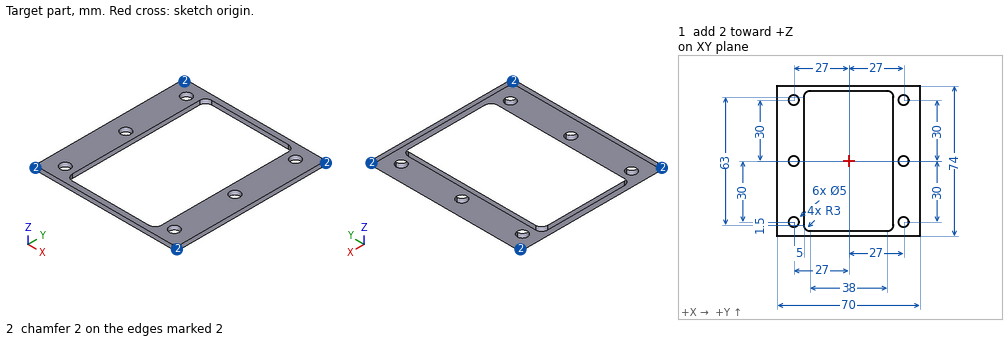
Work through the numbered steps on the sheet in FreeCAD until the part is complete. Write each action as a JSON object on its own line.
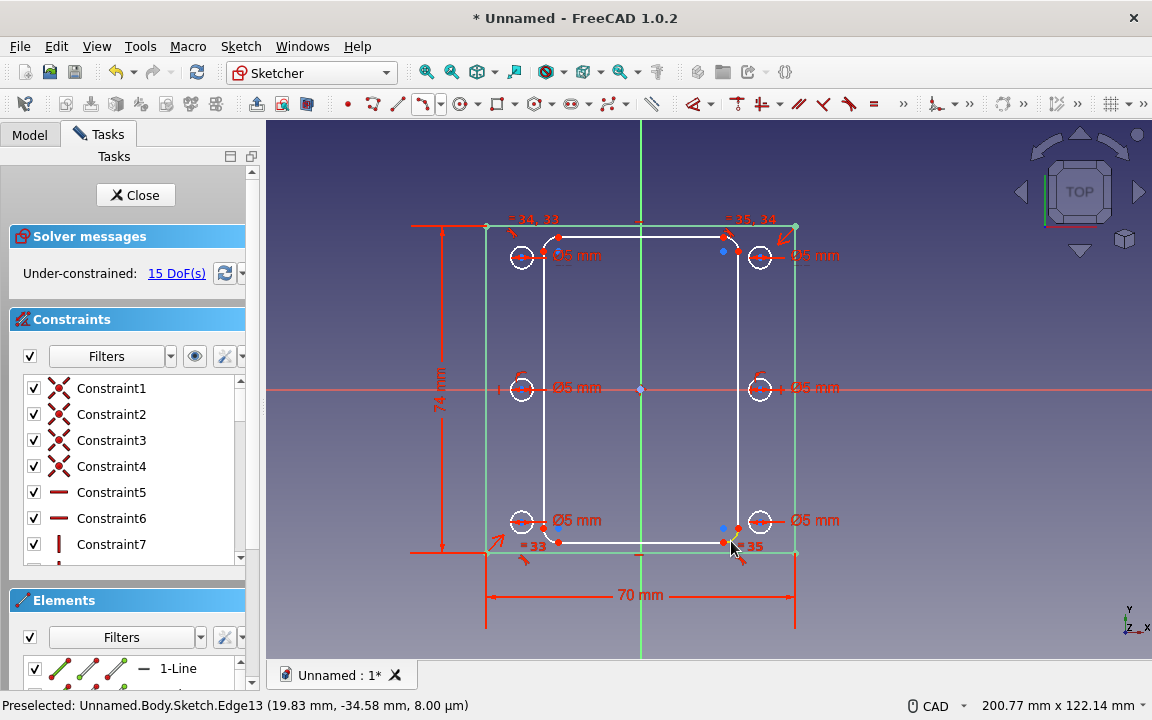
{"action": "left_click", "coordinate": [522, 522]}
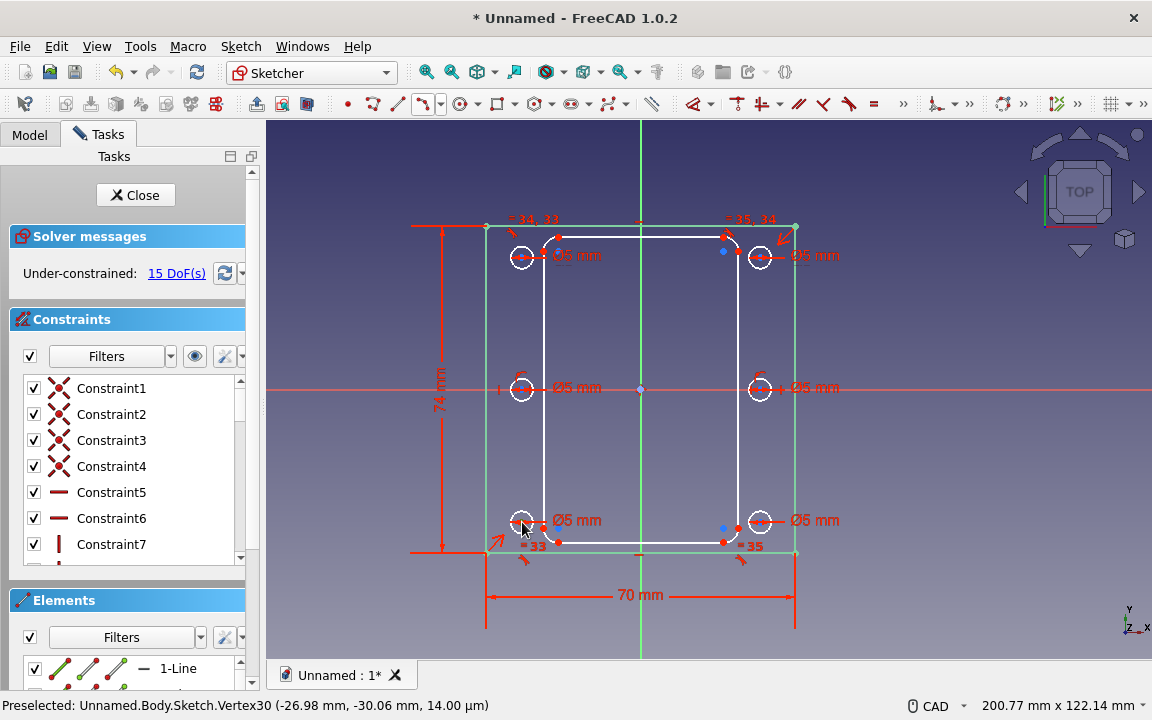
{"action": "left_click", "coordinate": [522, 390]}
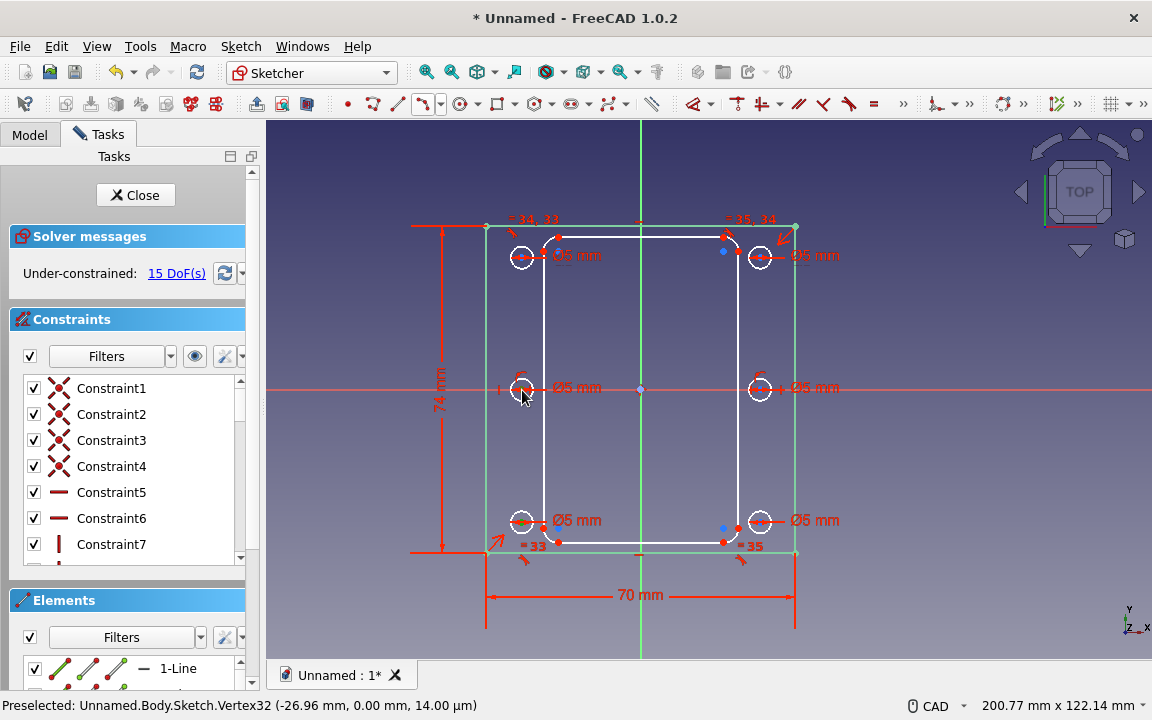
{"action": "key", "text": "v"}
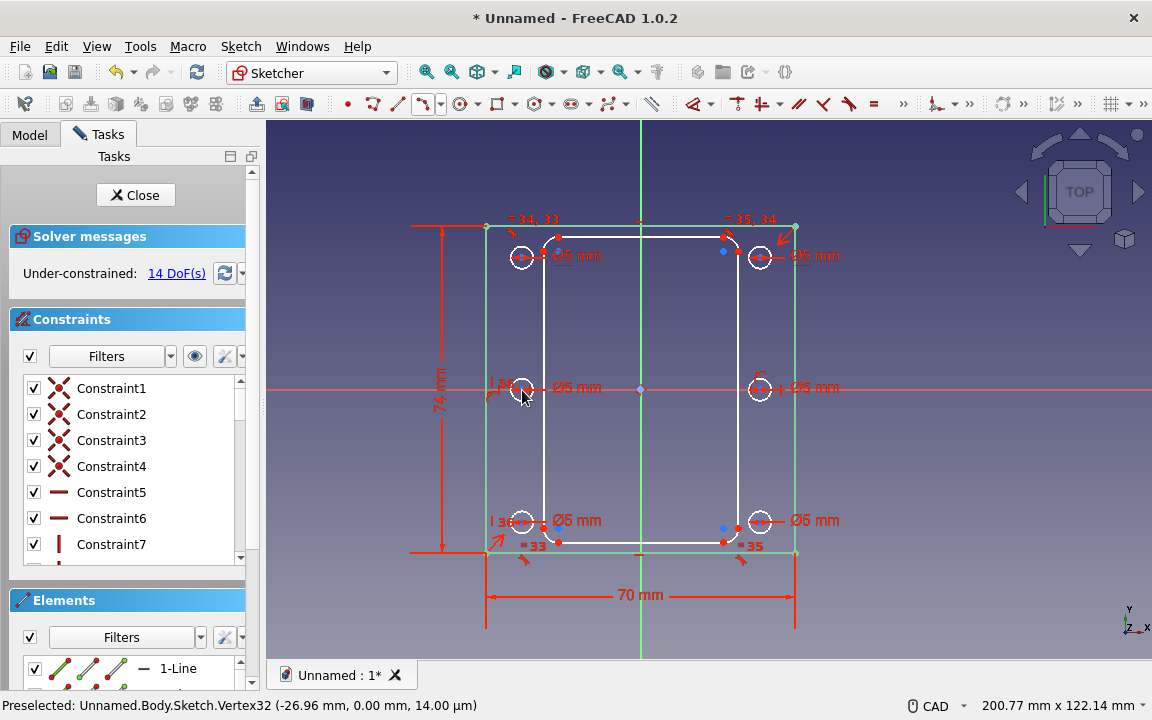
{"action": "left_click", "coordinate": [760, 522]}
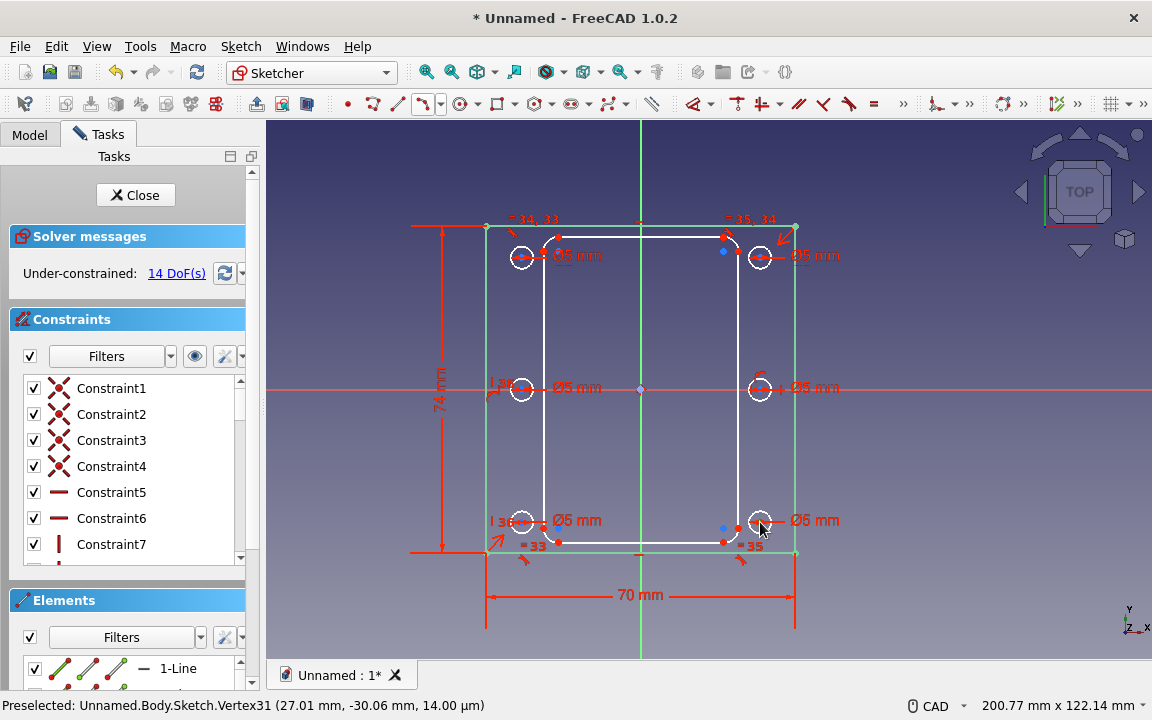
{"action": "left_click", "coordinate": [760, 390]}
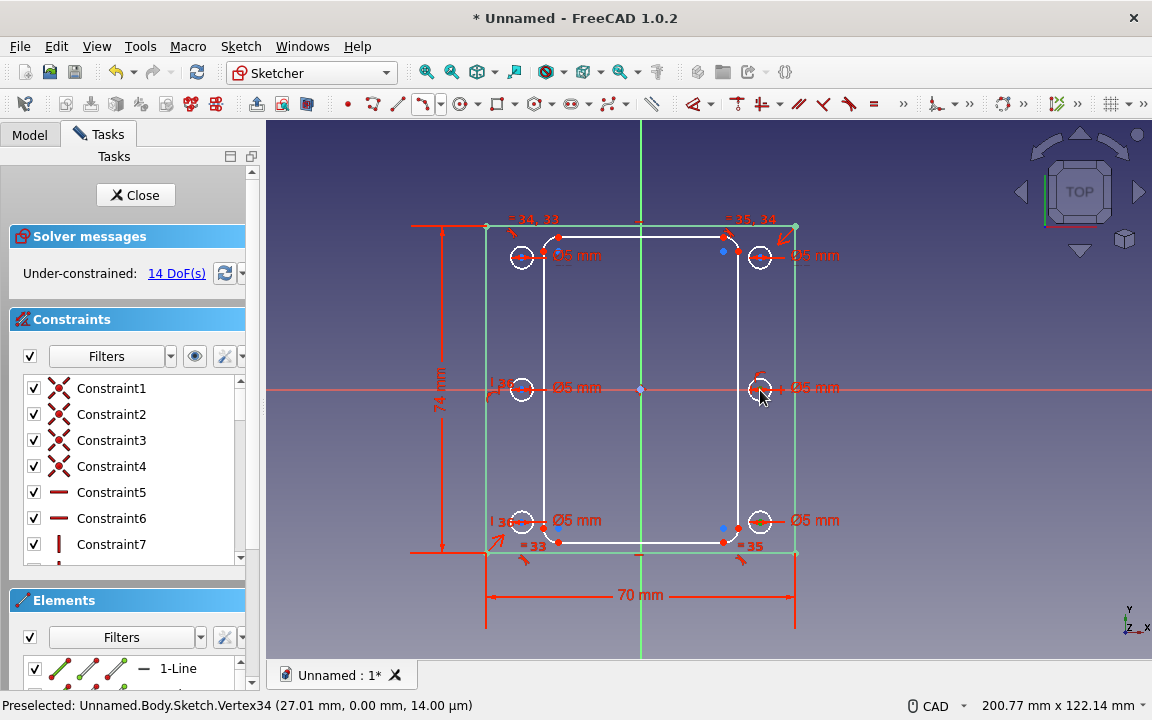
{"action": "key", "text": "v"}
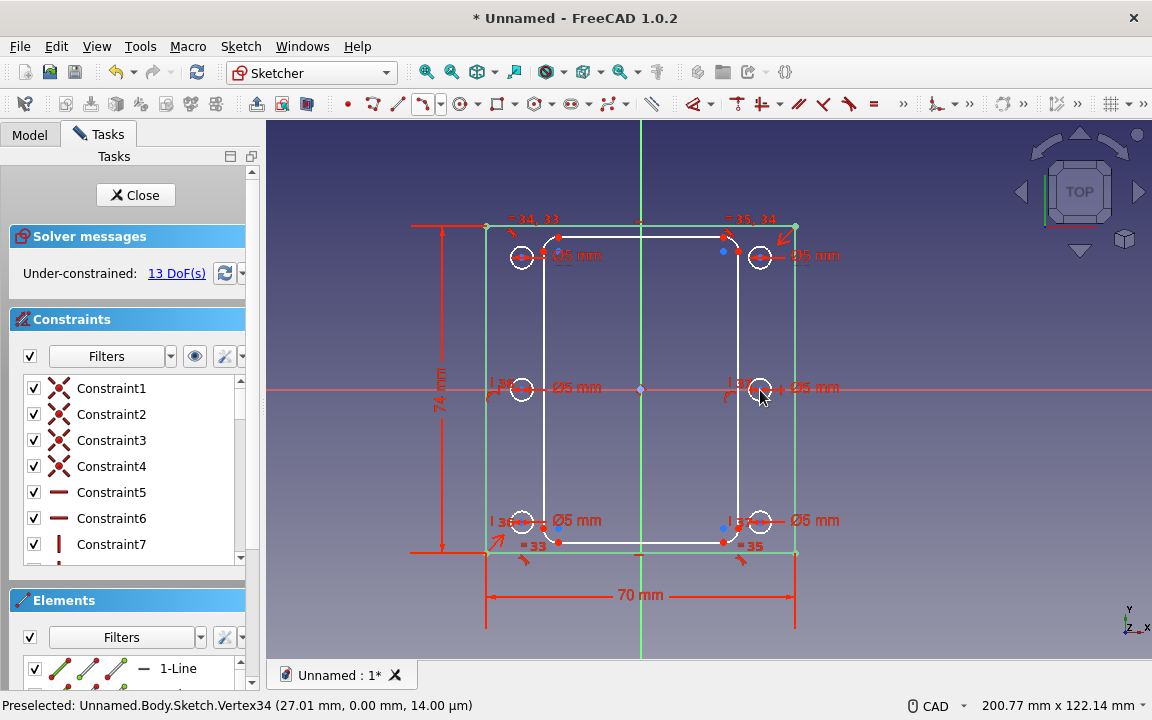
{"action": "key", "text": "d"}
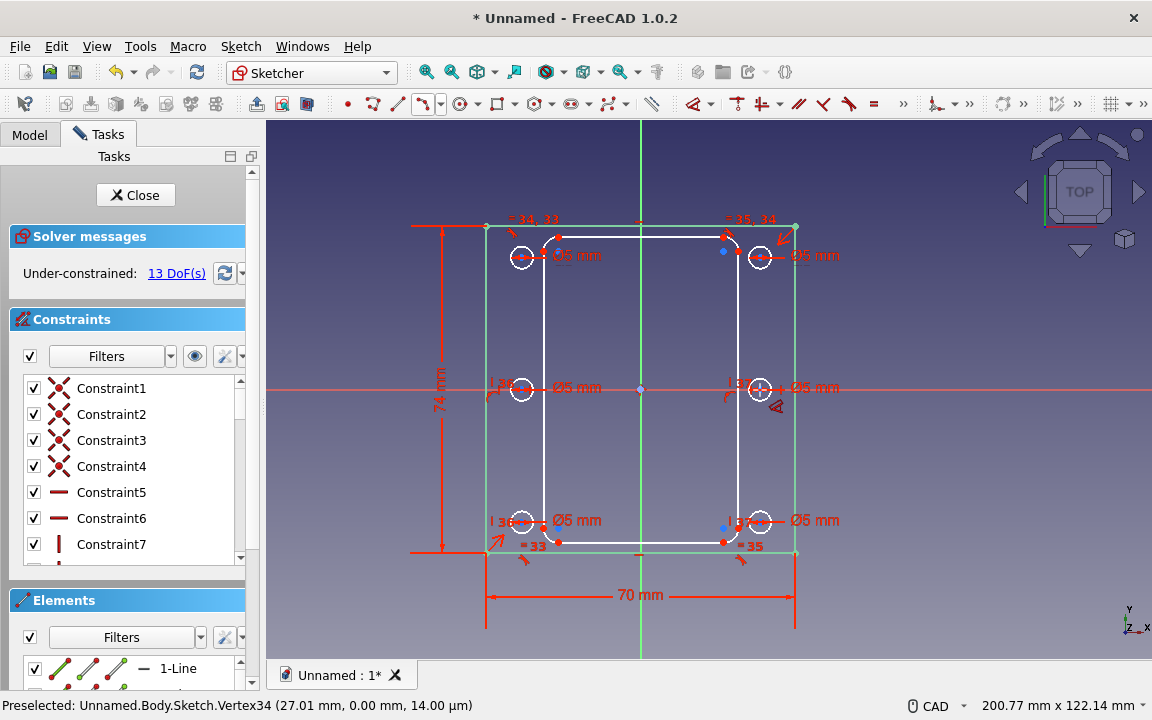
{"action": "scroll", "coordinate": [548, 538], "scroll_direction": "up", "scroll_amount": 6}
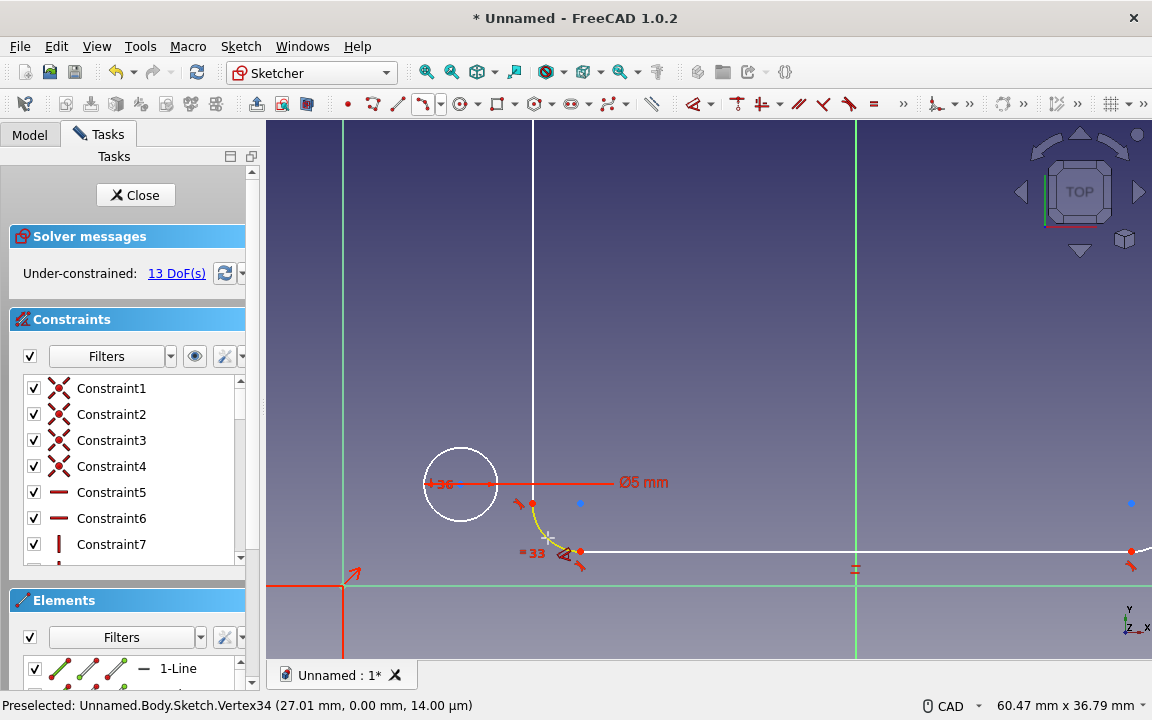
{"action": "left_click", "coordinate": [547, 538]}
{"action": "left_click", "coordinate": [525, 561]}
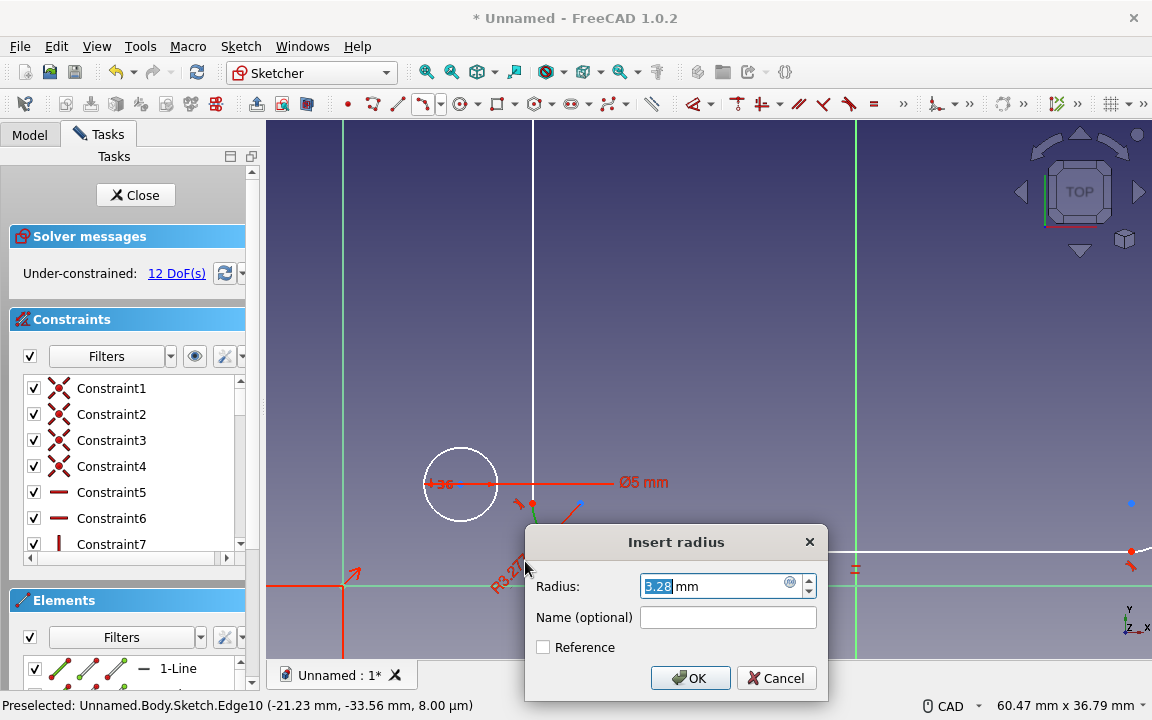
{"action": "type", "text": "3"}
{"action": "key", "text": "Return"}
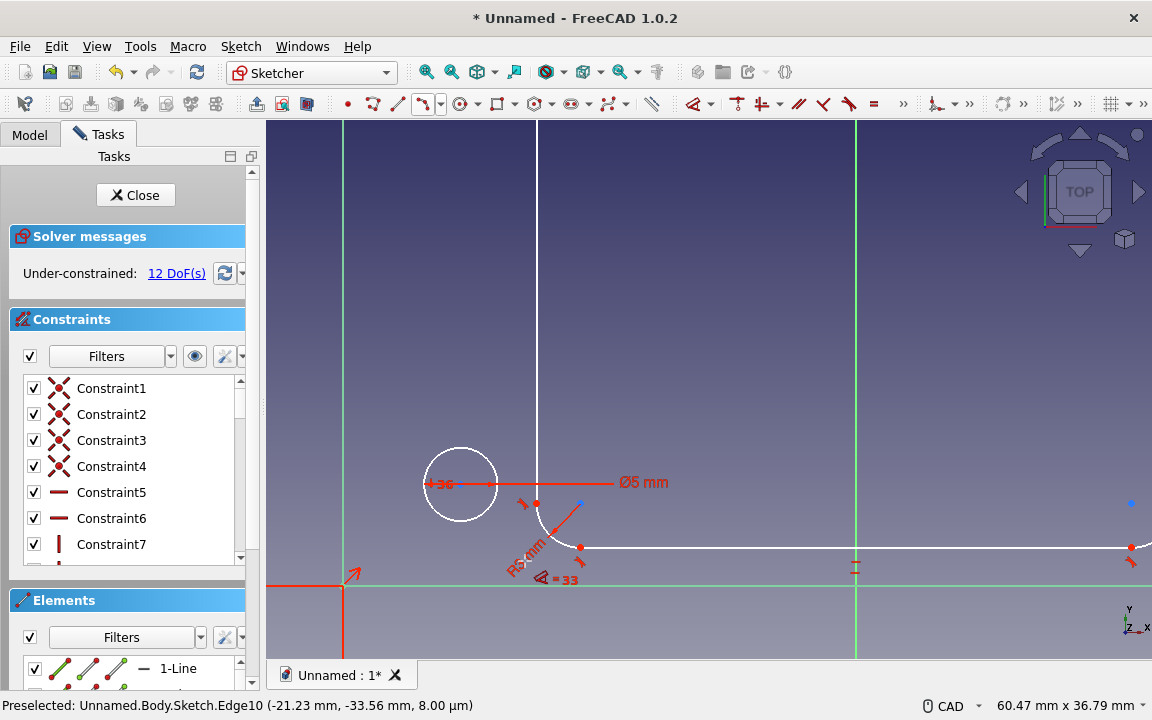
{"action": "left_click", "coordinate": [966, 548]}
{"action": "left_click", "coordinate": [784, 514]}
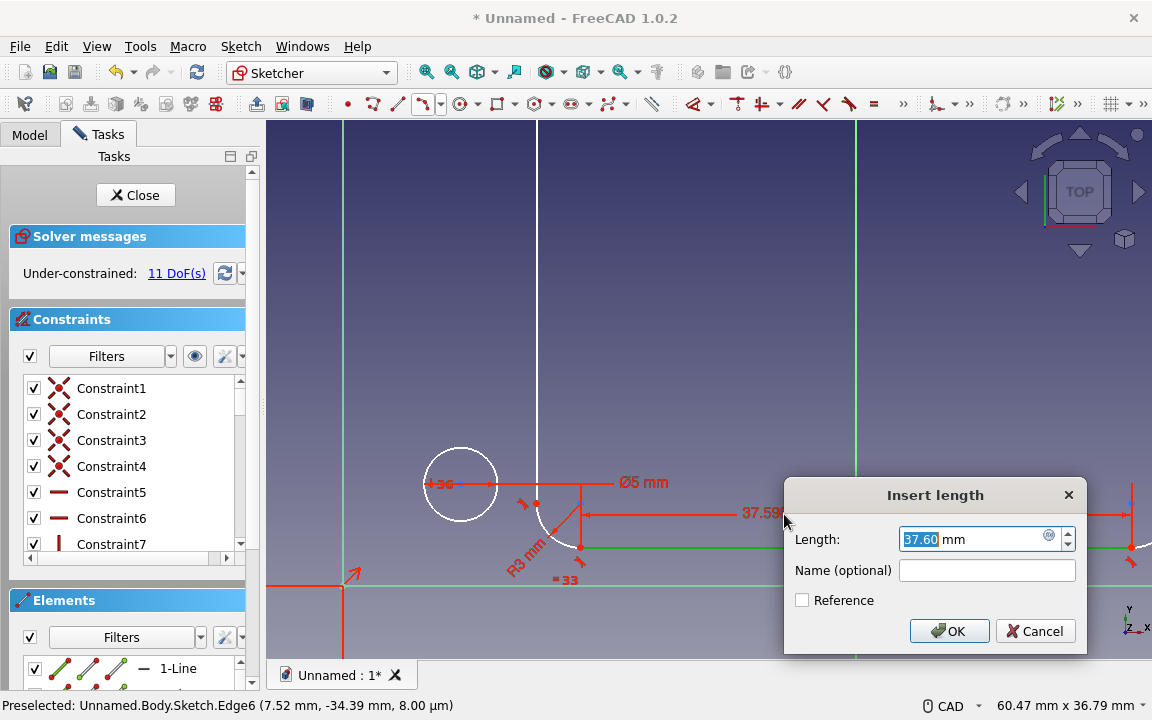
{"action": "type", "text": "38"}
{"action": "key", "text": "Return"}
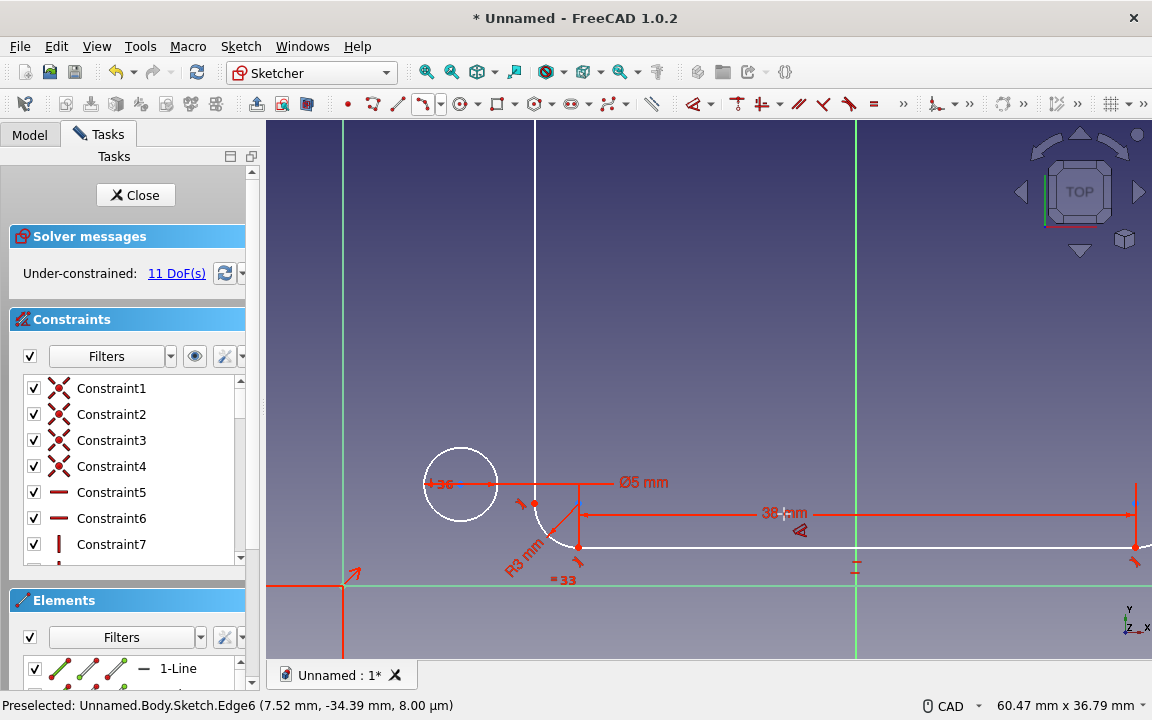
{"action": "left_click", "coordinate": [535, 228]}
{"action": "left_click", "coordinate": [501, 326]}